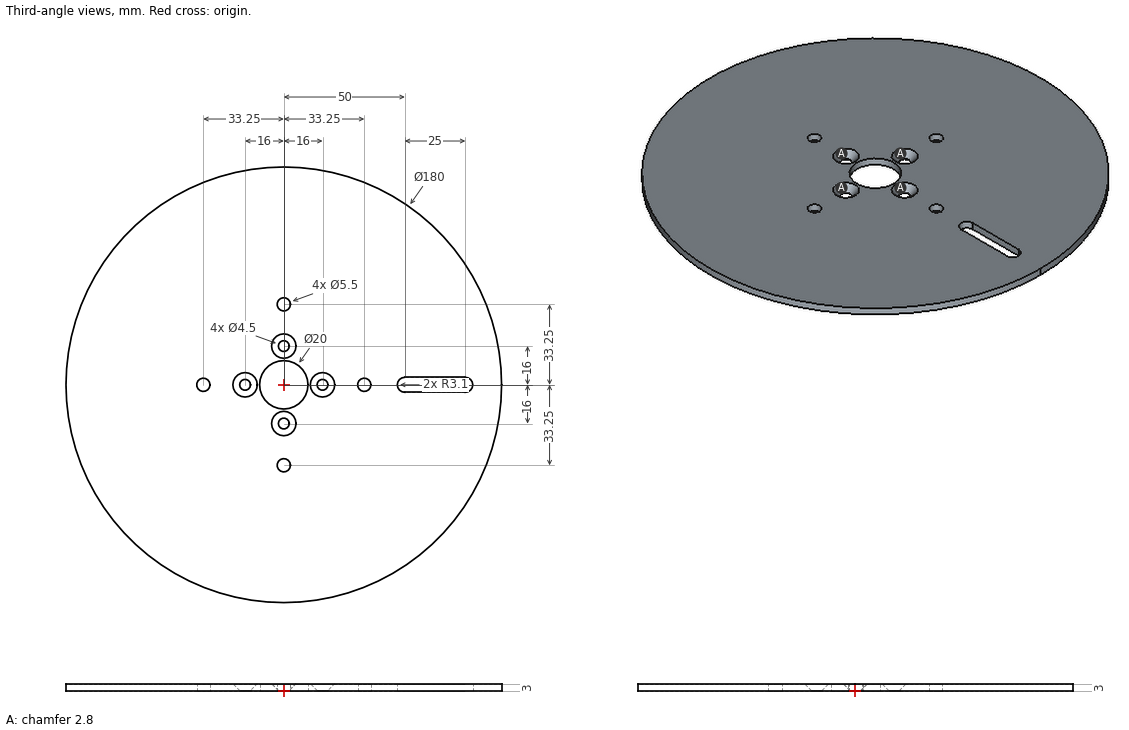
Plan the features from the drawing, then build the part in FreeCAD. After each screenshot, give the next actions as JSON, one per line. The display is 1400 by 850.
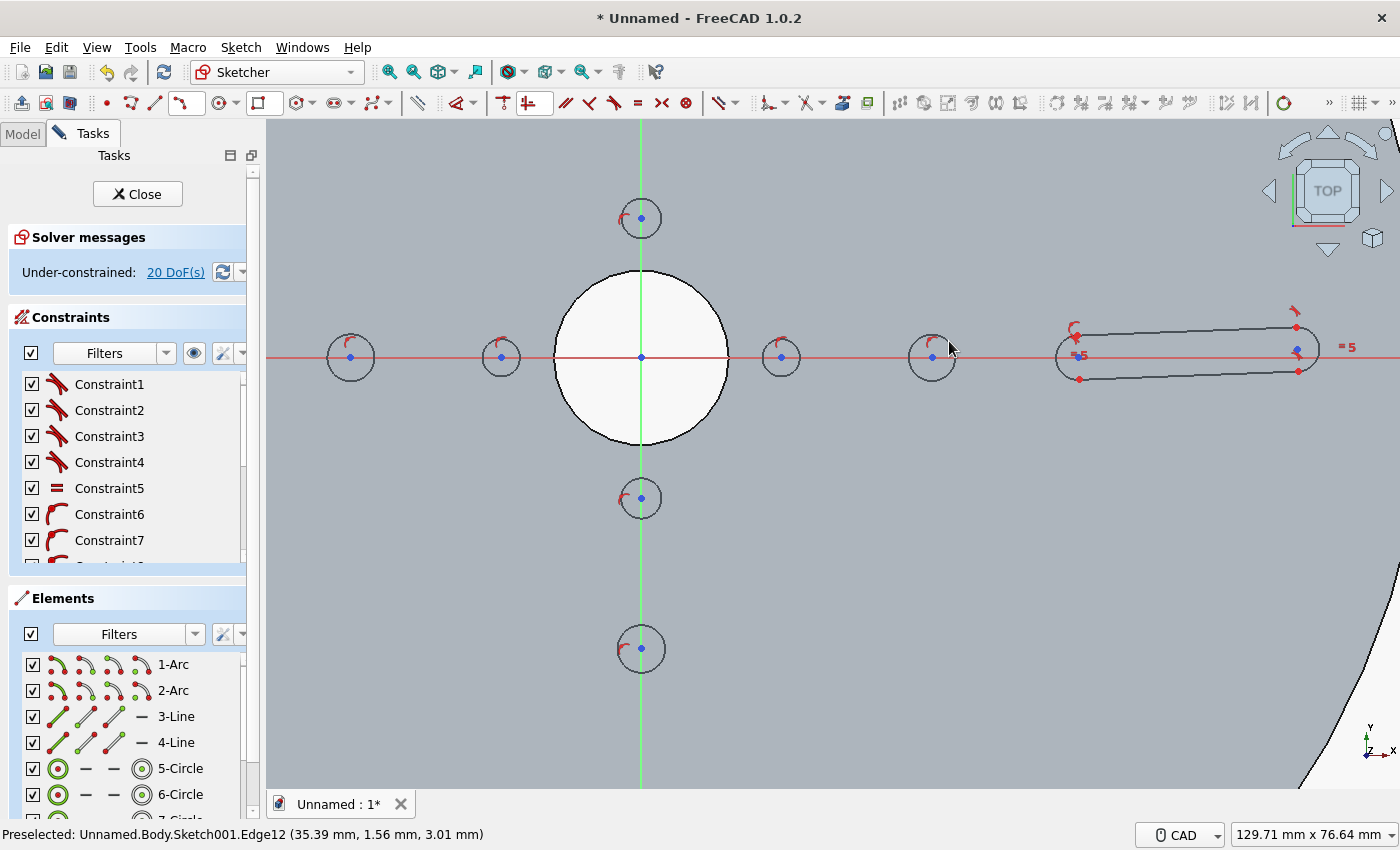
{"action": "left_click", "coordinate": [1143, 333]}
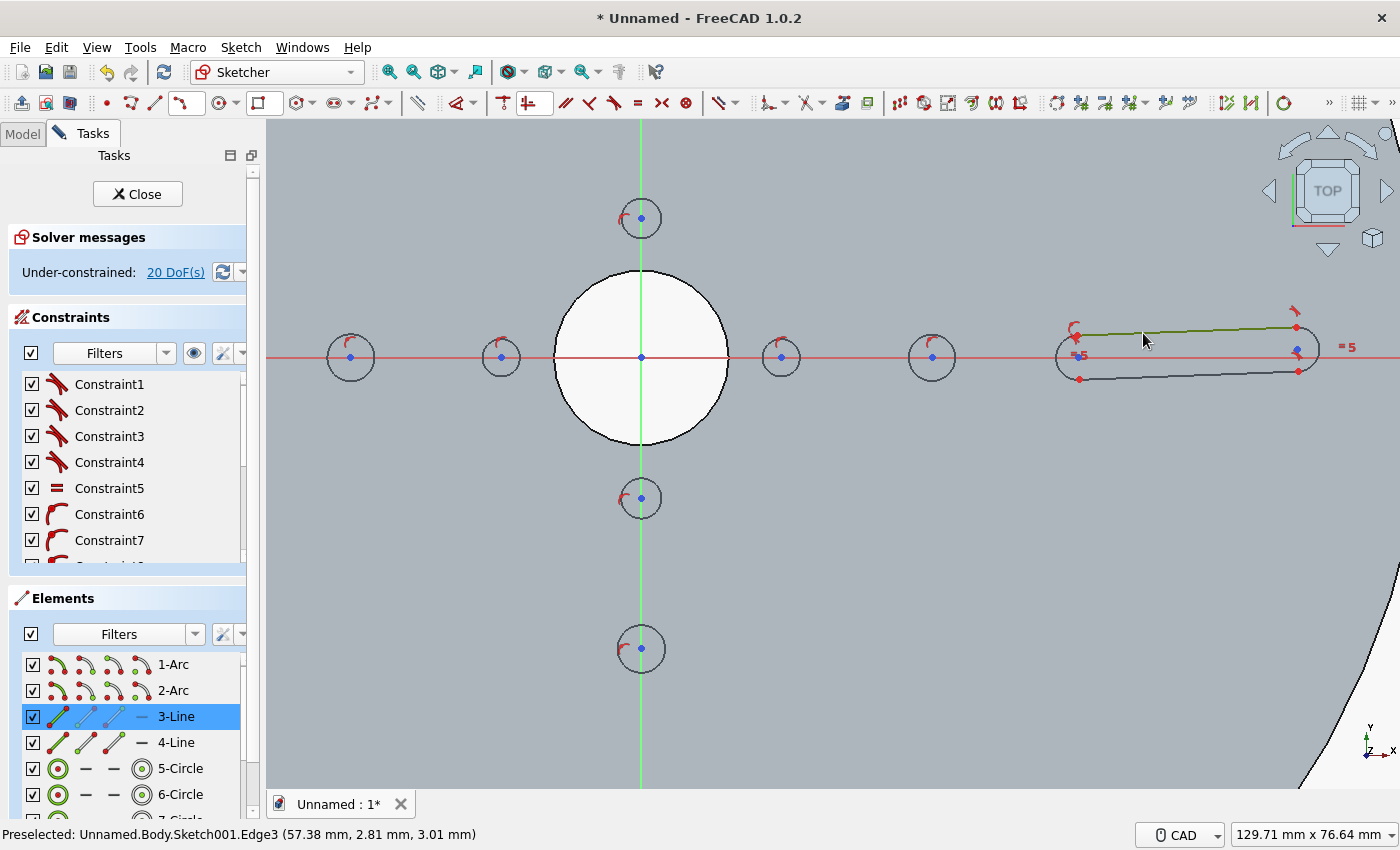
{"action": "left_click", "coordinate": [548, 104]}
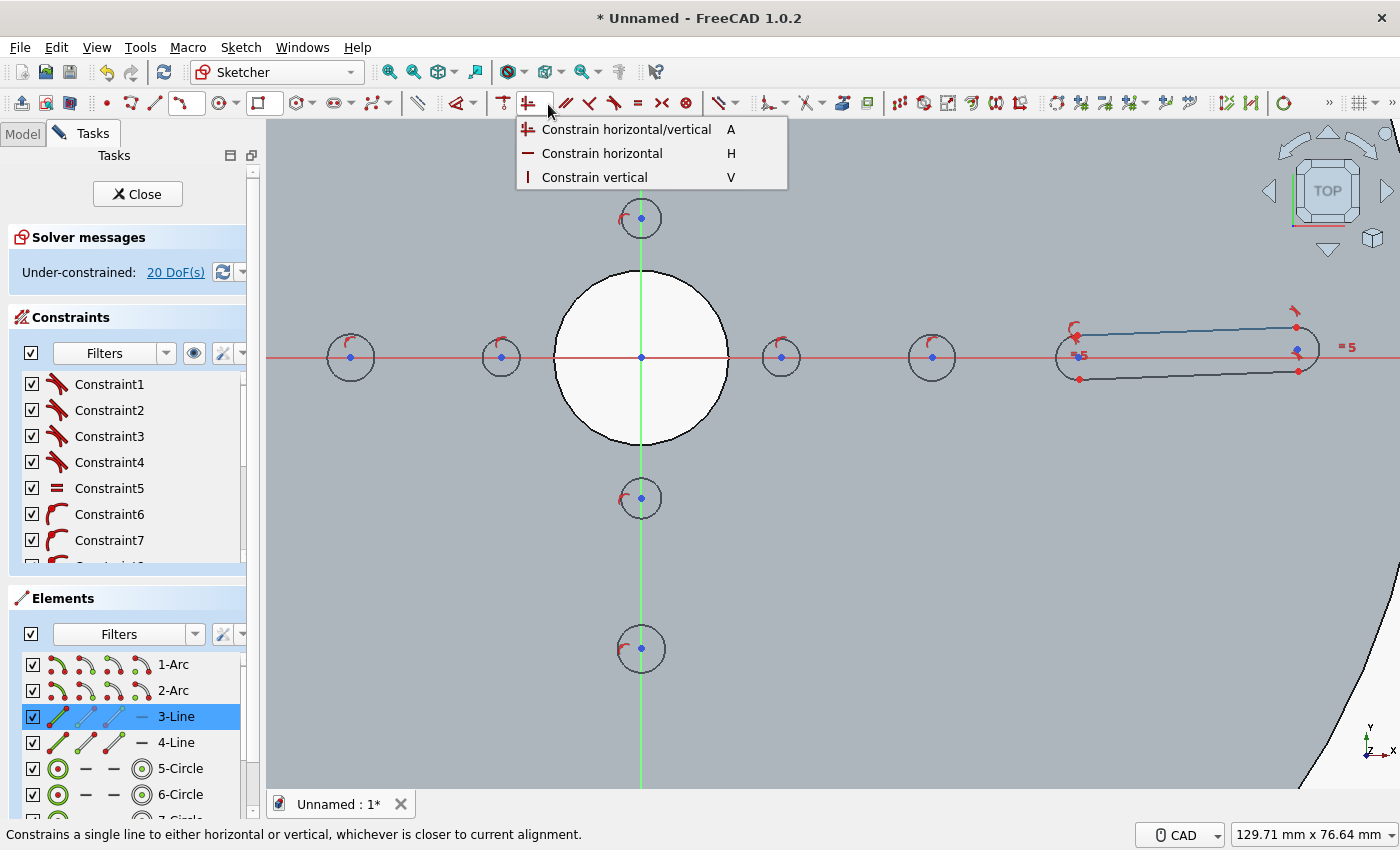
{"action": "left_click", "coordinate": [652, 153]}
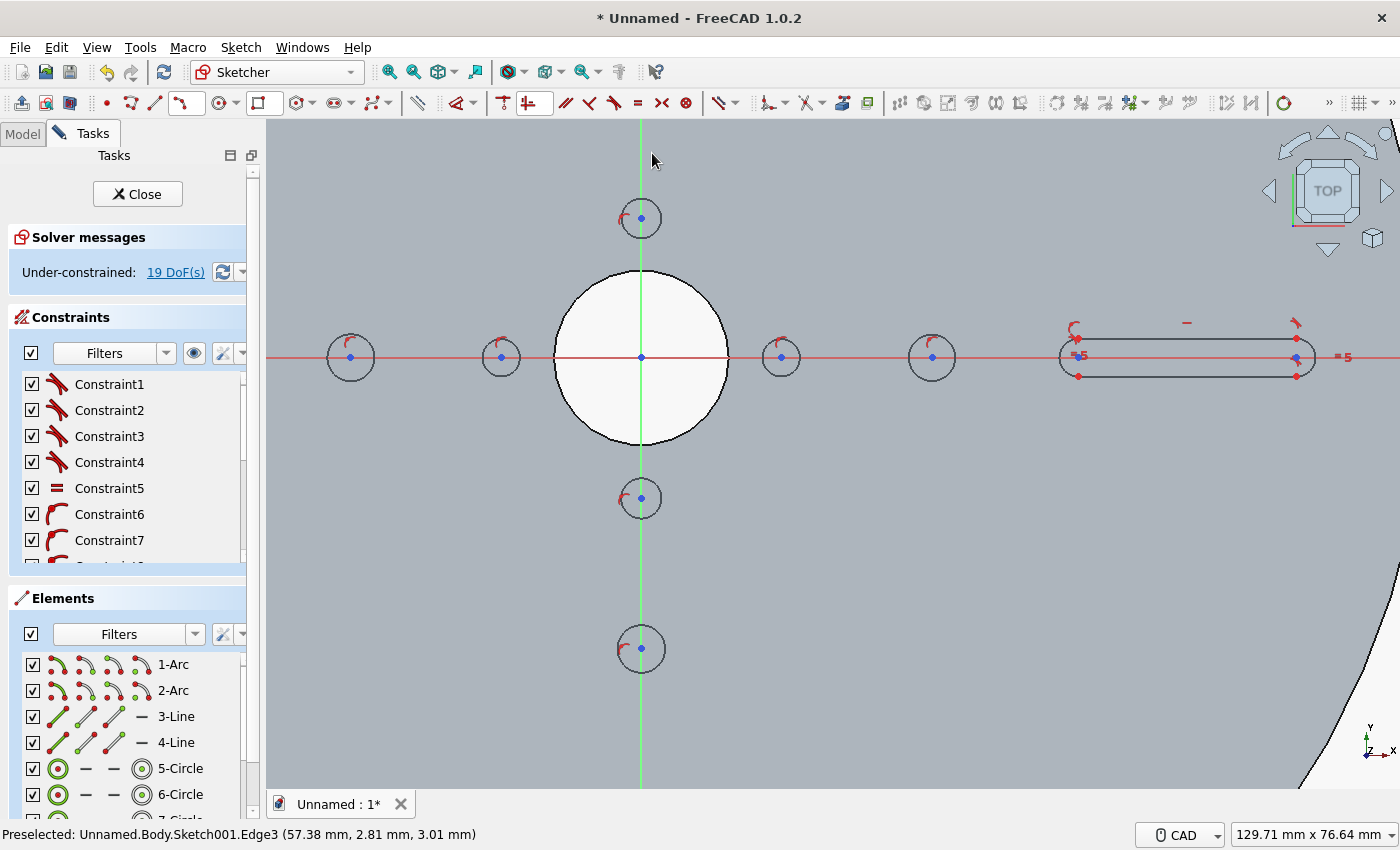
{"action": "left_click", "coordinate": [655, 204]}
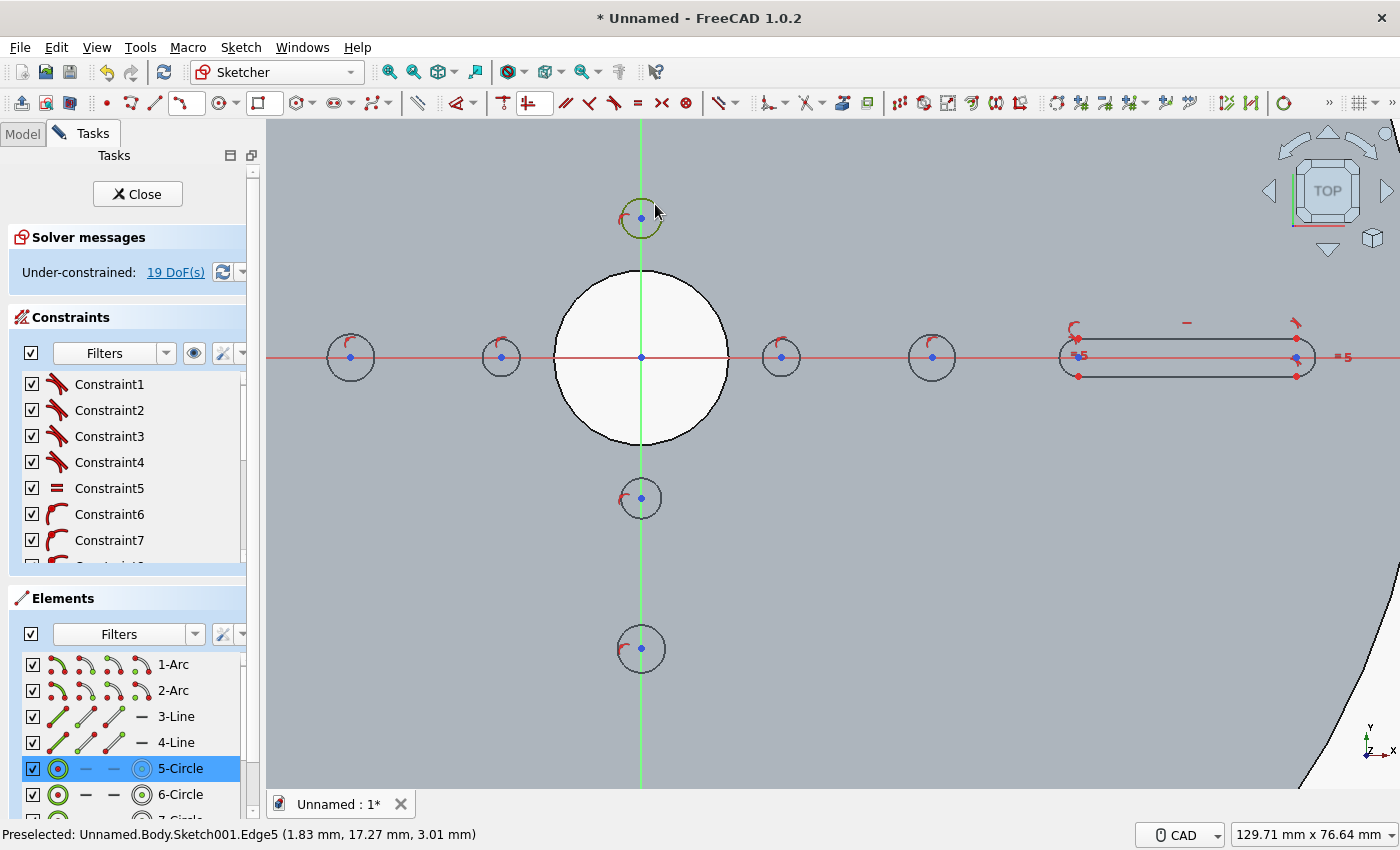
{"action": "left_click", "coordinate": [514, 345]}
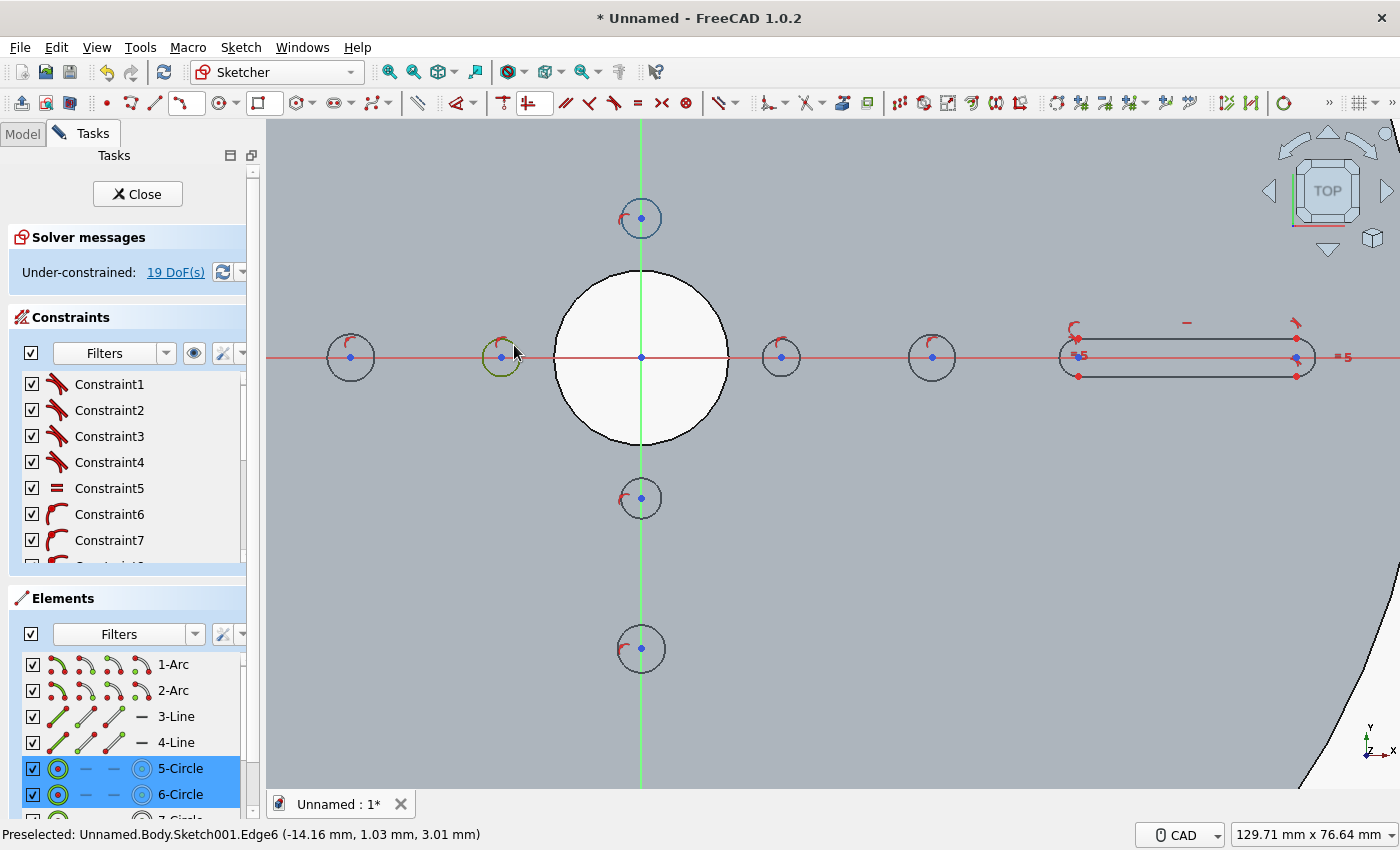
{"action": "left_click", "coordinate": [656, 484]}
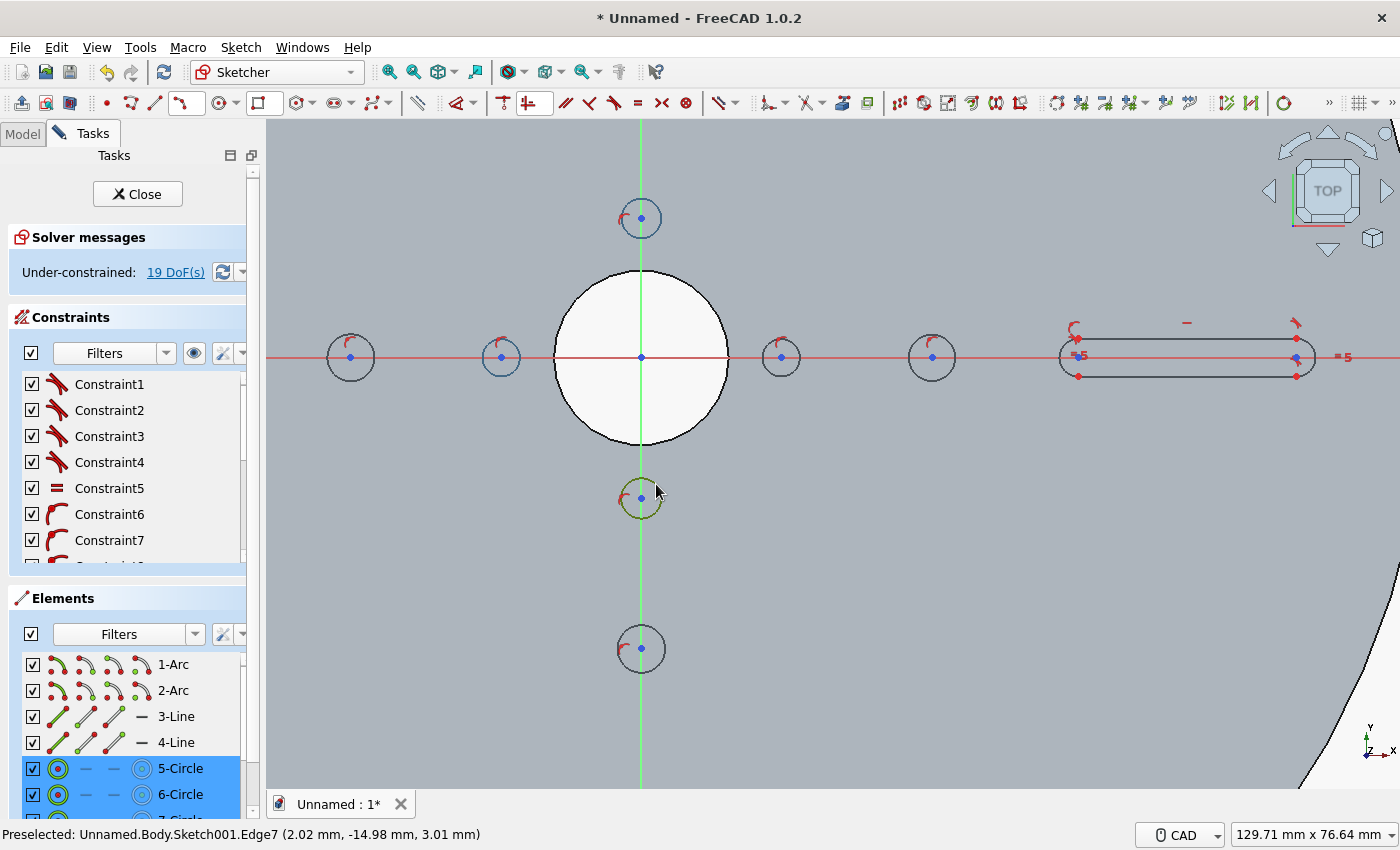
{"action": "left_click", "coordinate": [794, 345]}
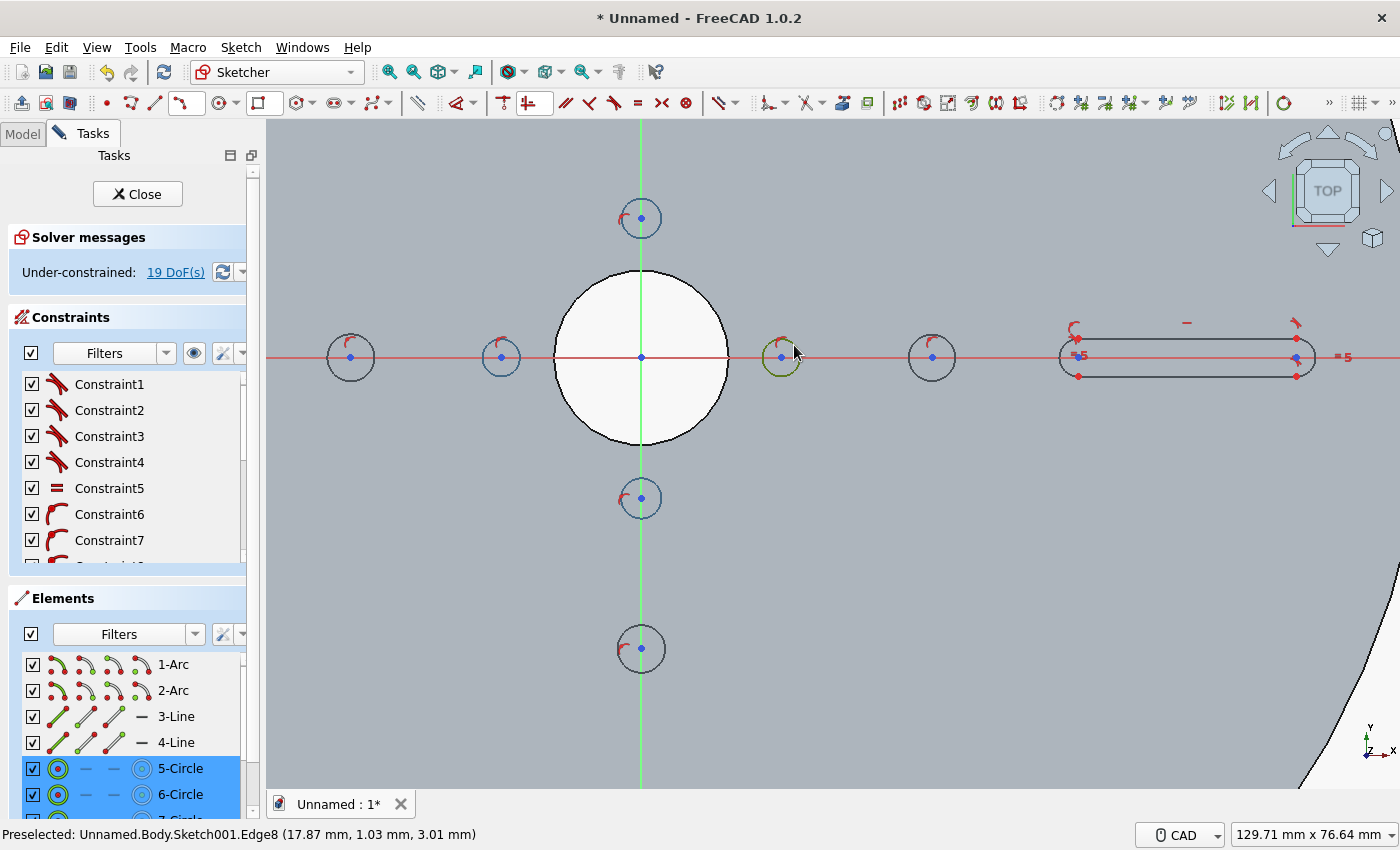
{"action": "left_click", "coordinate": [638, 104]}